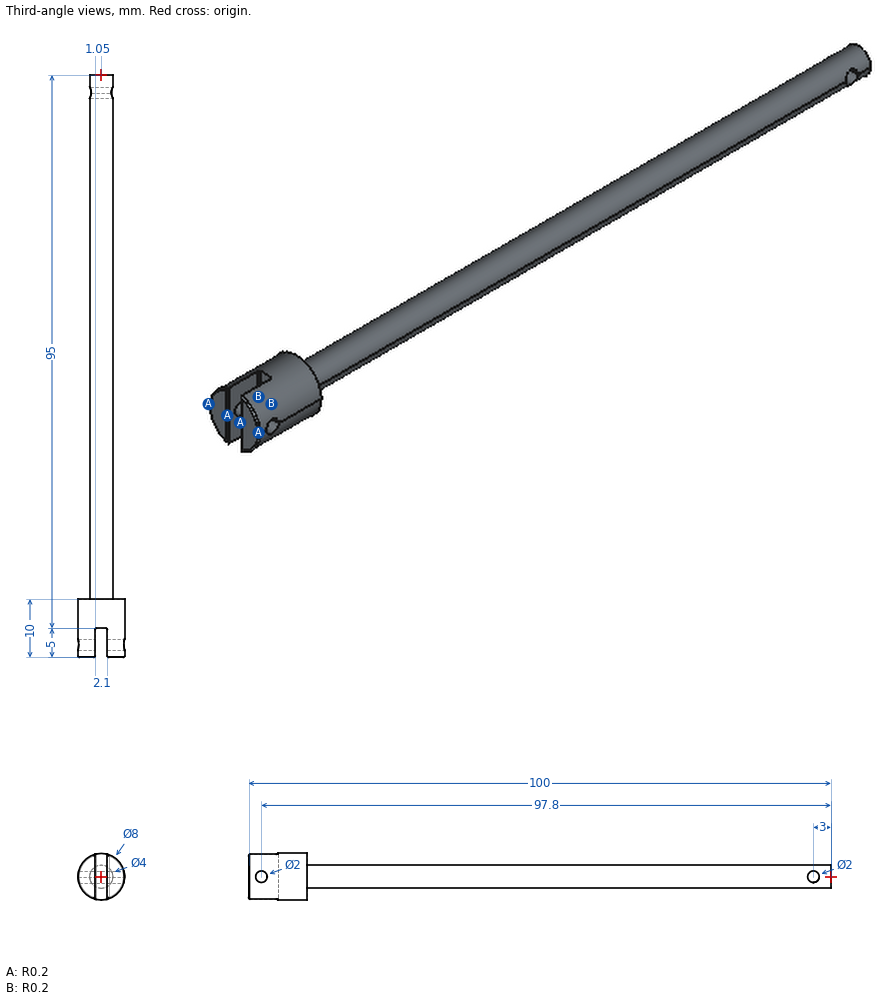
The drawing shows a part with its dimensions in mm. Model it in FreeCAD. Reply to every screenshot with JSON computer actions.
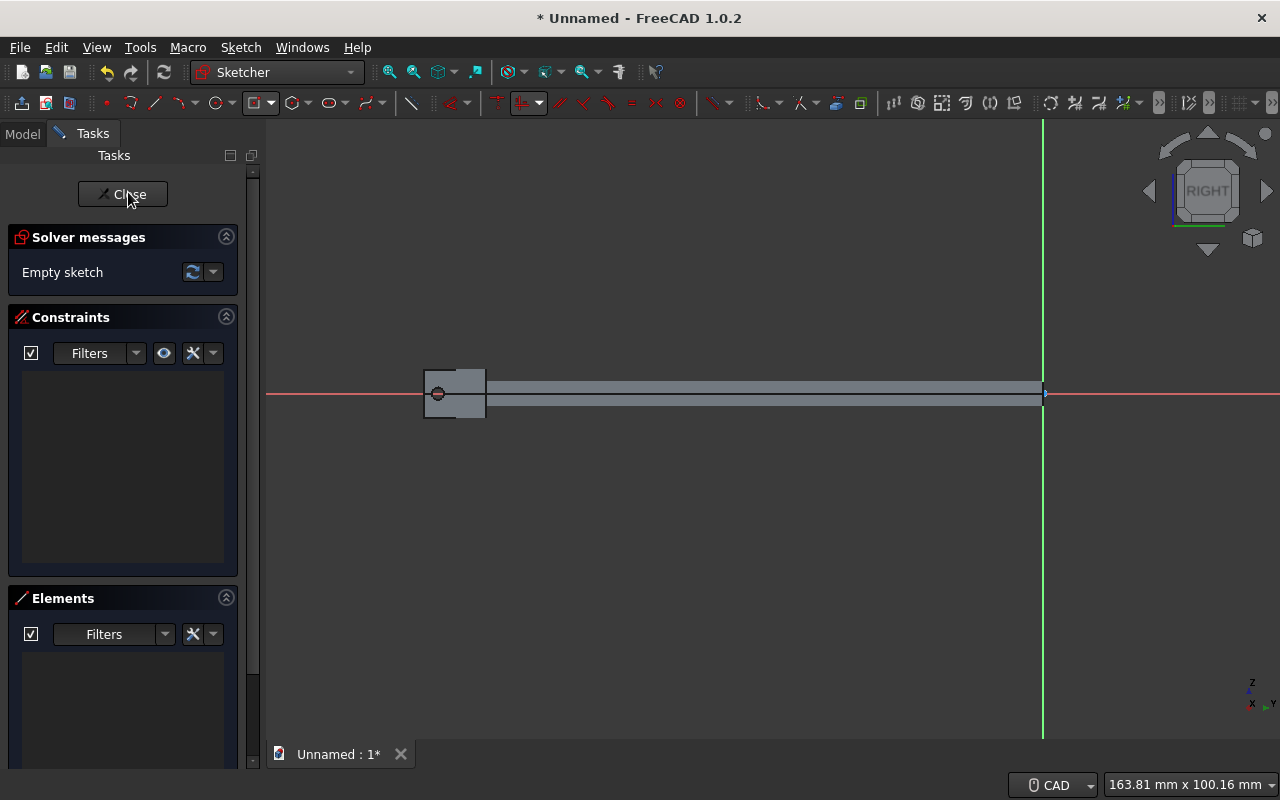
{"action": "left_click", "coordinate": [70, 104]}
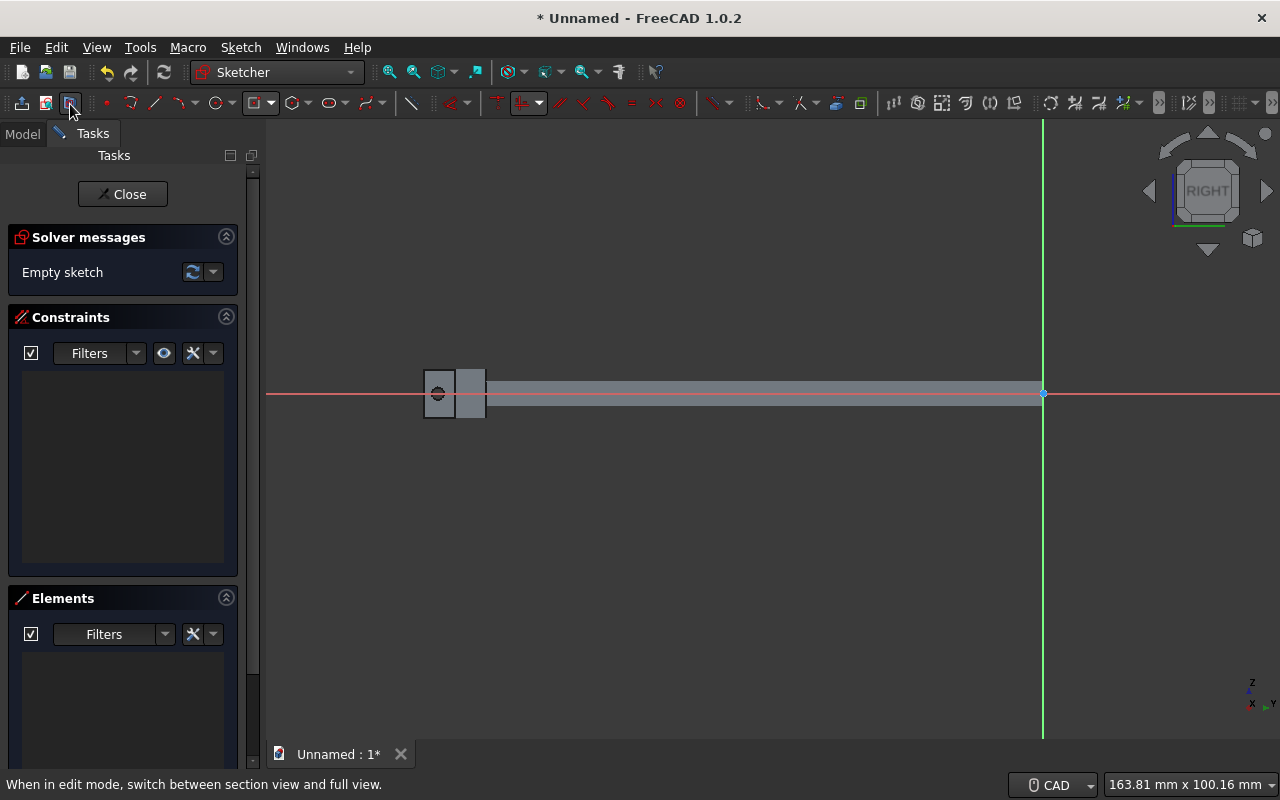
{"action": "scroll", "coordinate": [1048, 392], "scroll_direction": "up", "scroll_amount": 15}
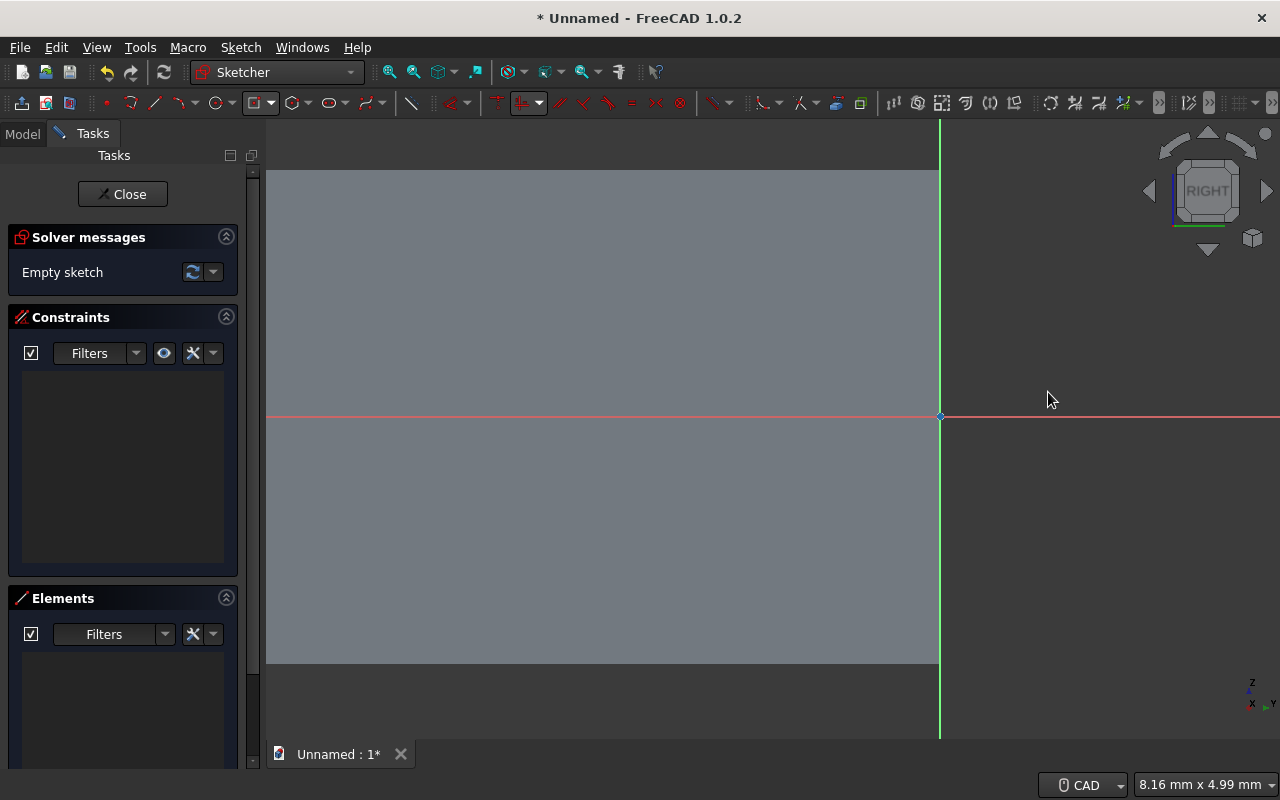
{"action": "left_click", "coordinate": [216, 104]}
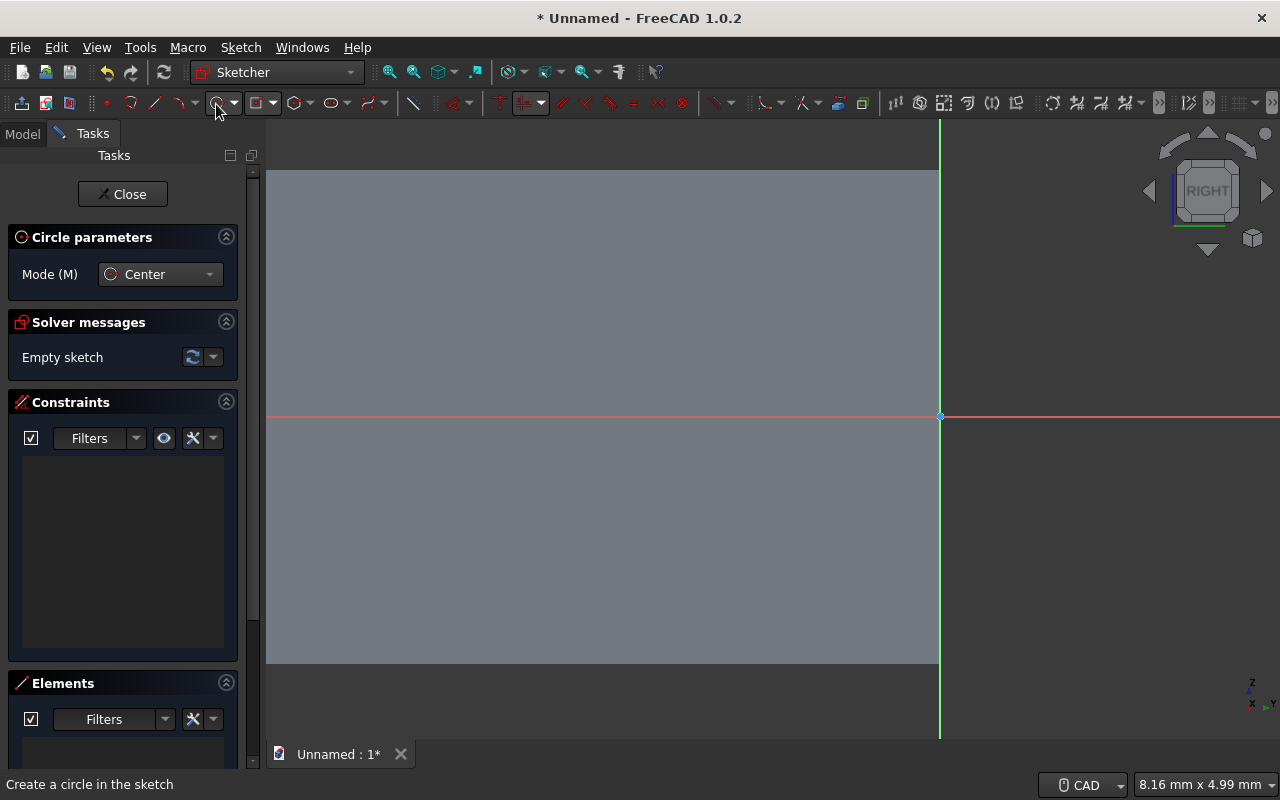
{"action": "left_click", "coordinate": [567, 417]}
{"action": "left_click", "coordinate": [655, 329]}
{"action": "key", "text": "Escape"}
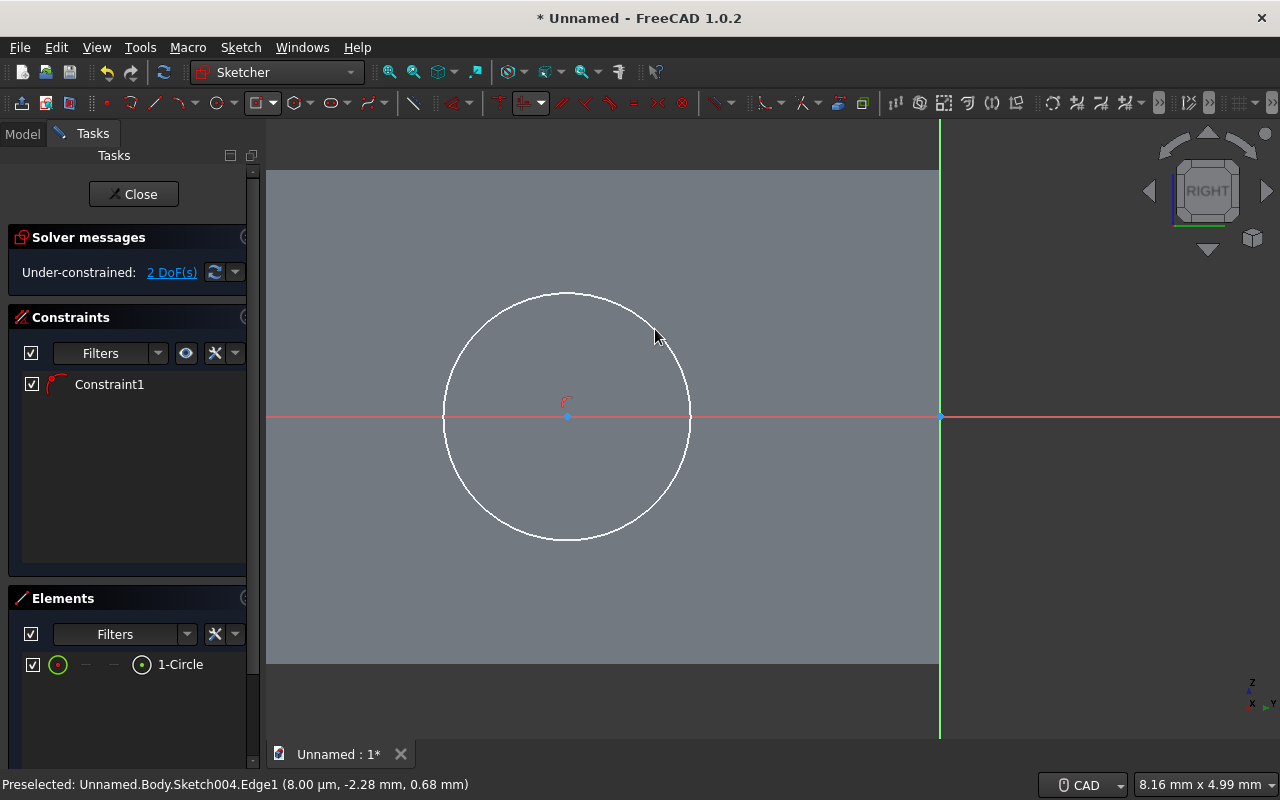
{"action": "left_click", "coordinate": [452, 104]}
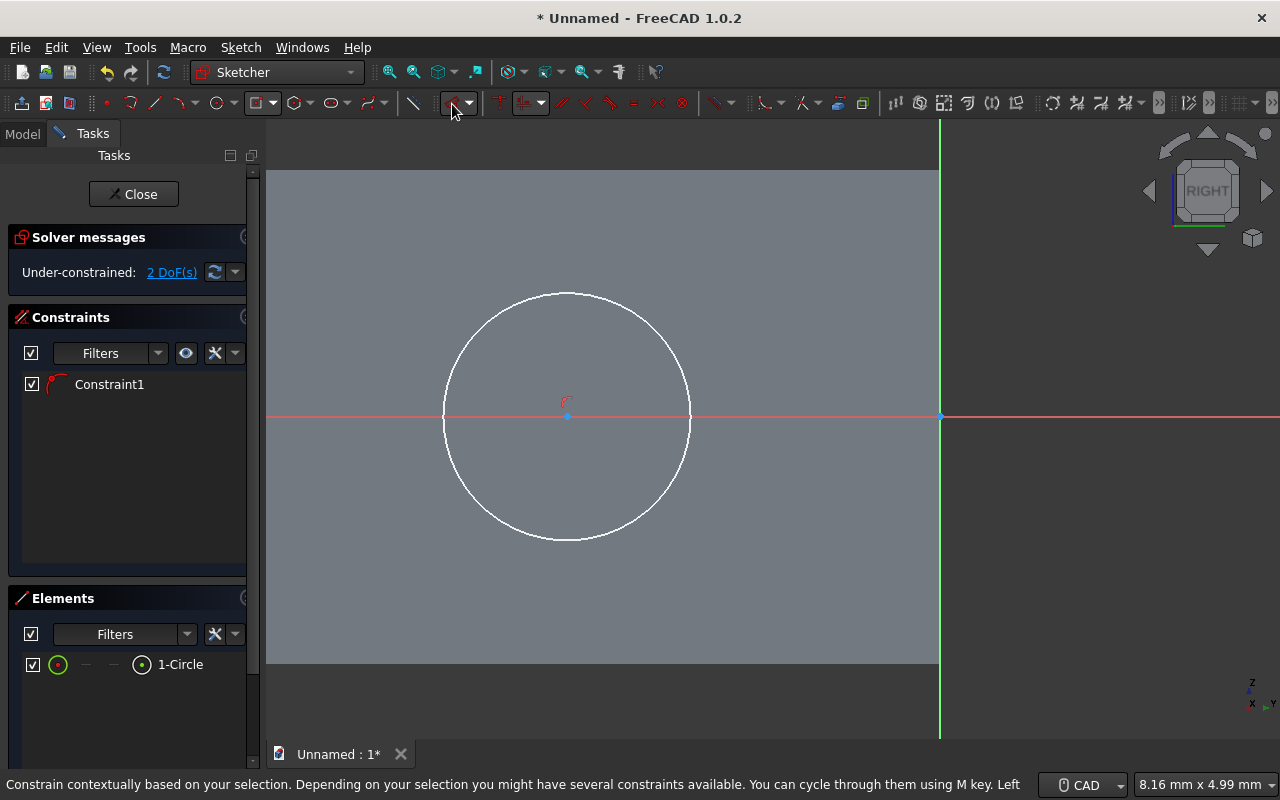
{"action": "left_click", "coordinate": [654, 329]}
{"action": "left_click", "coordinate": [677, 306]}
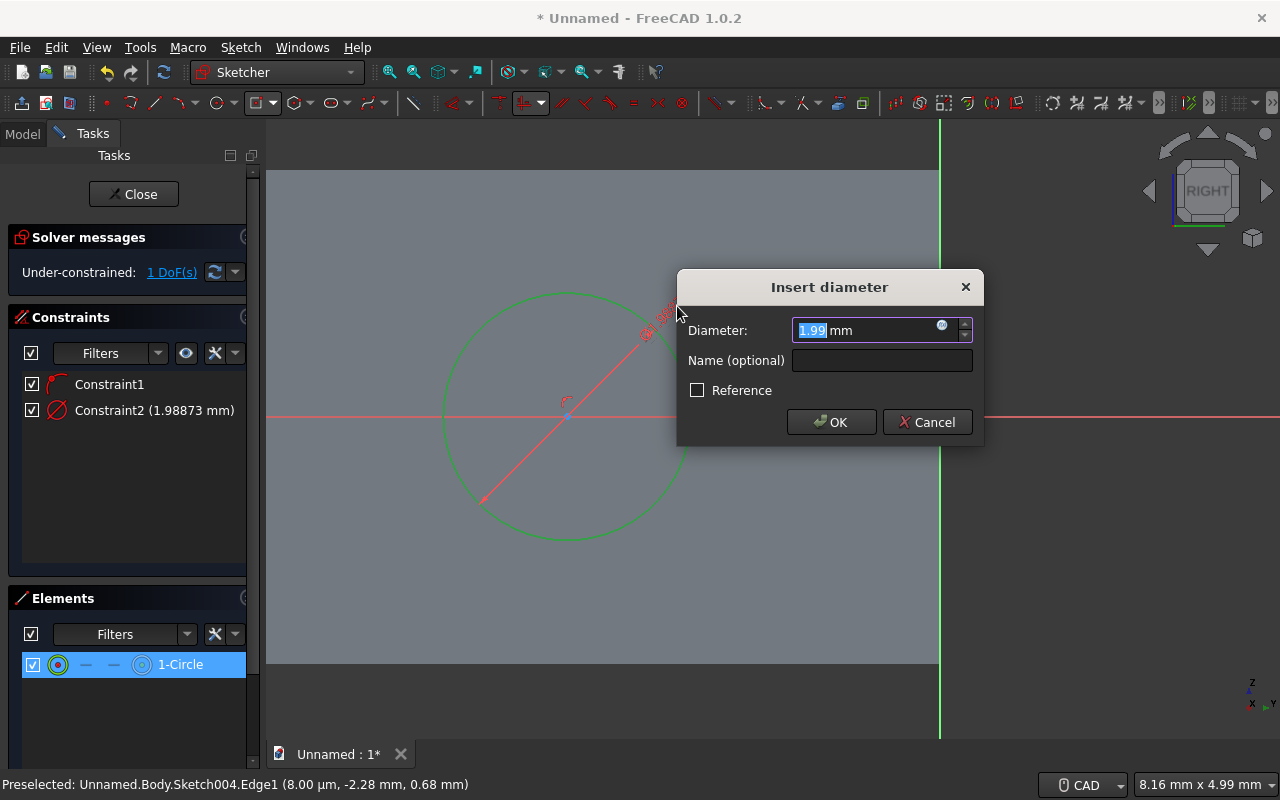
{"action": "type", "text": "2"}
{"action": "key", "text": "Return"}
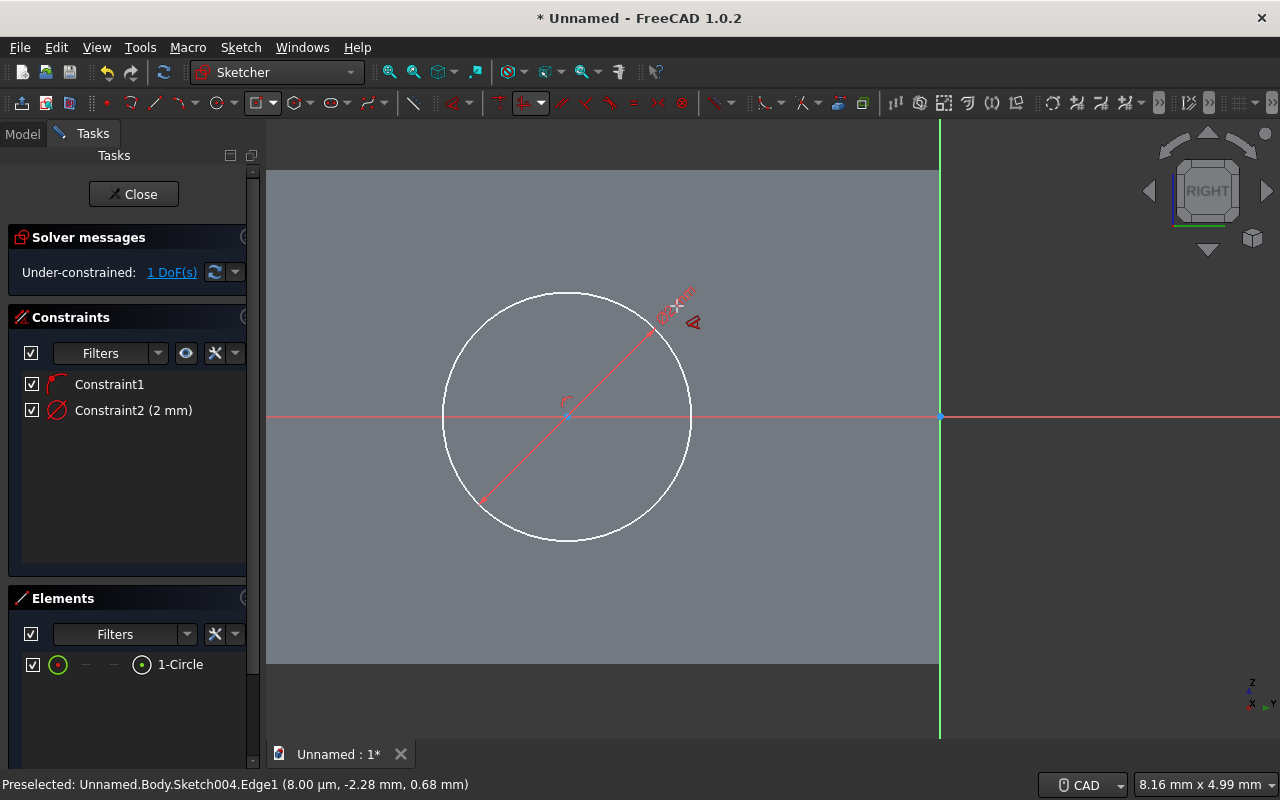
{"action": "left_click", "coordinate": [567, 417]}
{"action": "left_click", "coordinate": [754, 451]}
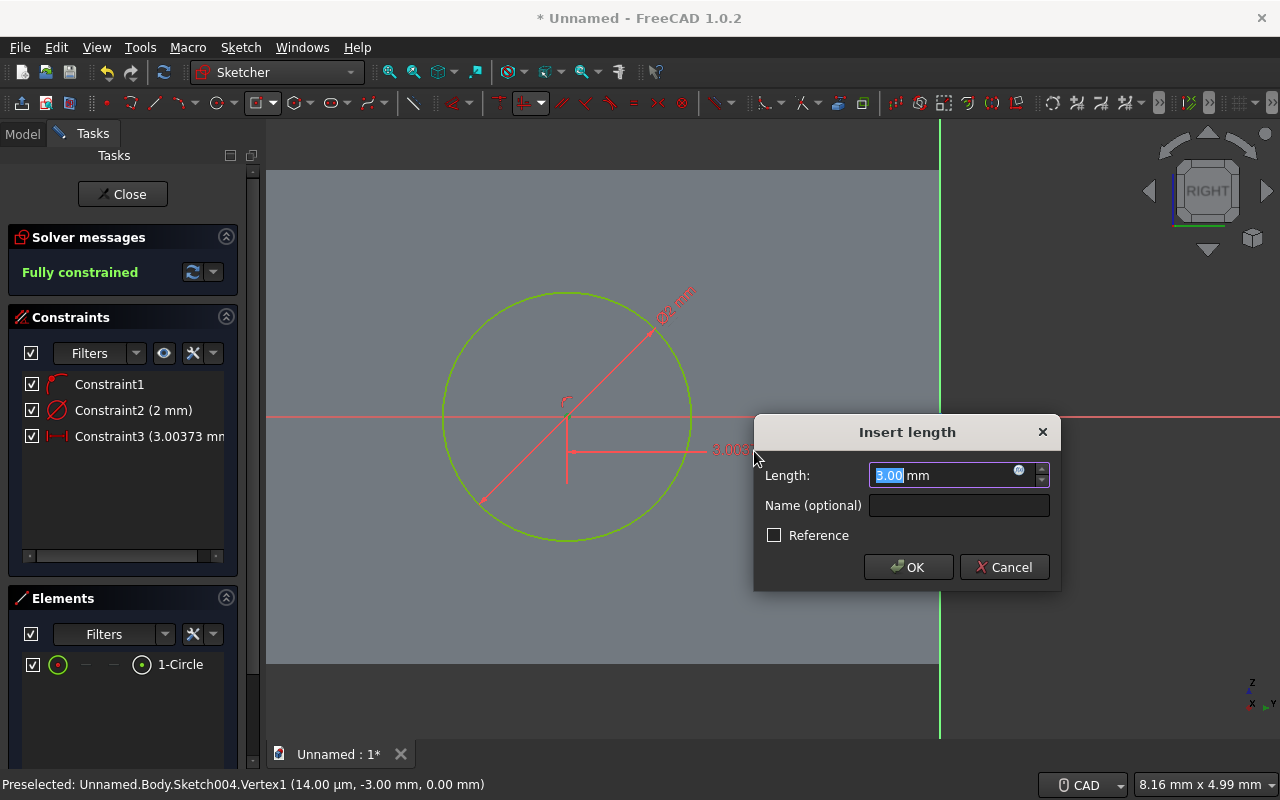
{"action": "type", "text": "3"}
{"action": "key", "text": "Return"}
{"action": "key", "text": "Escape"}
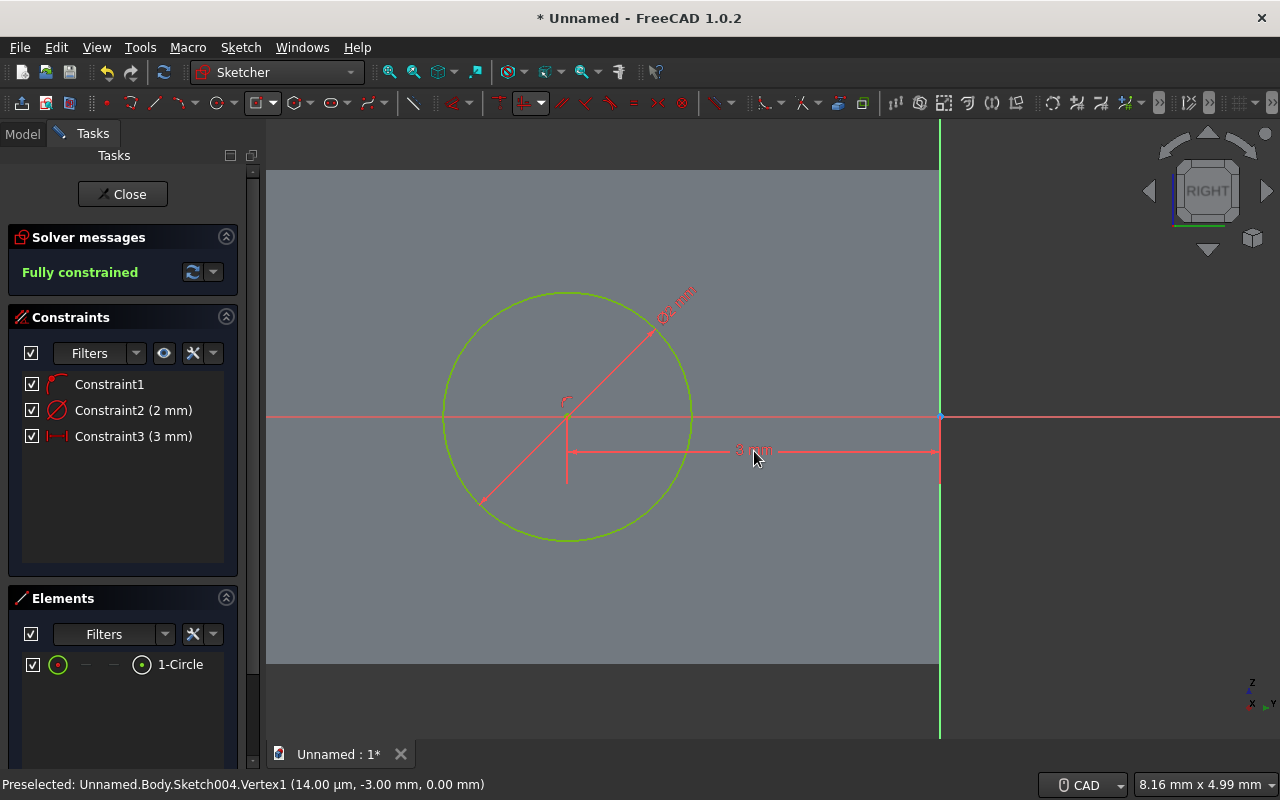
{"action": "left_click", "coordinate": [123, 194]}